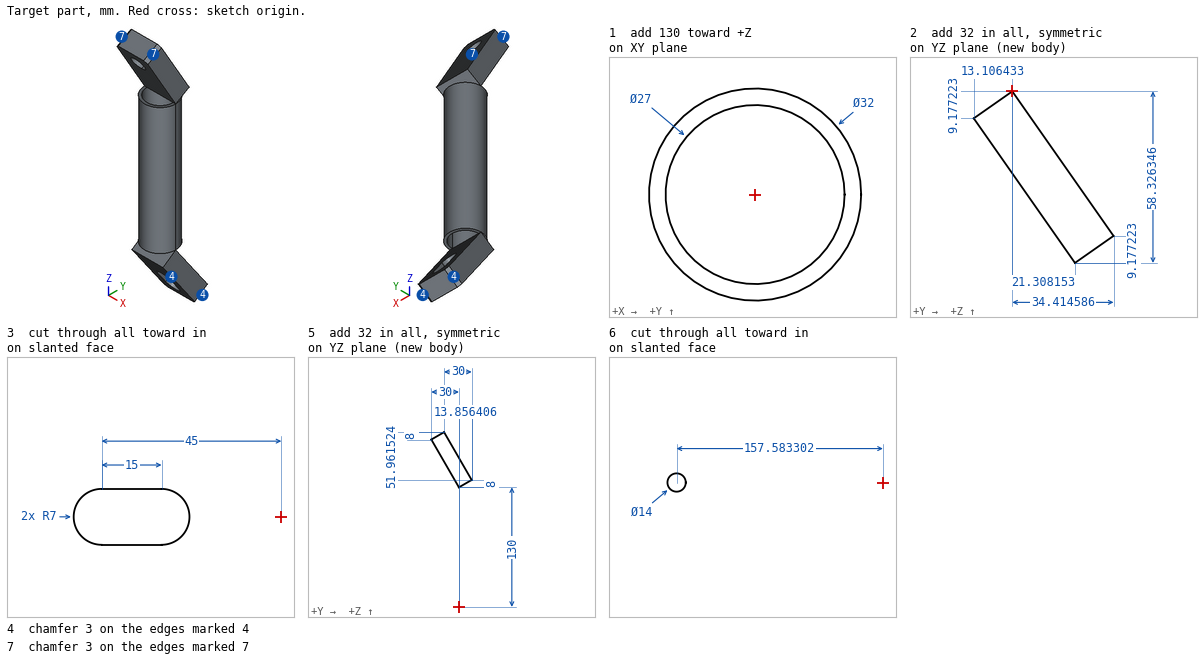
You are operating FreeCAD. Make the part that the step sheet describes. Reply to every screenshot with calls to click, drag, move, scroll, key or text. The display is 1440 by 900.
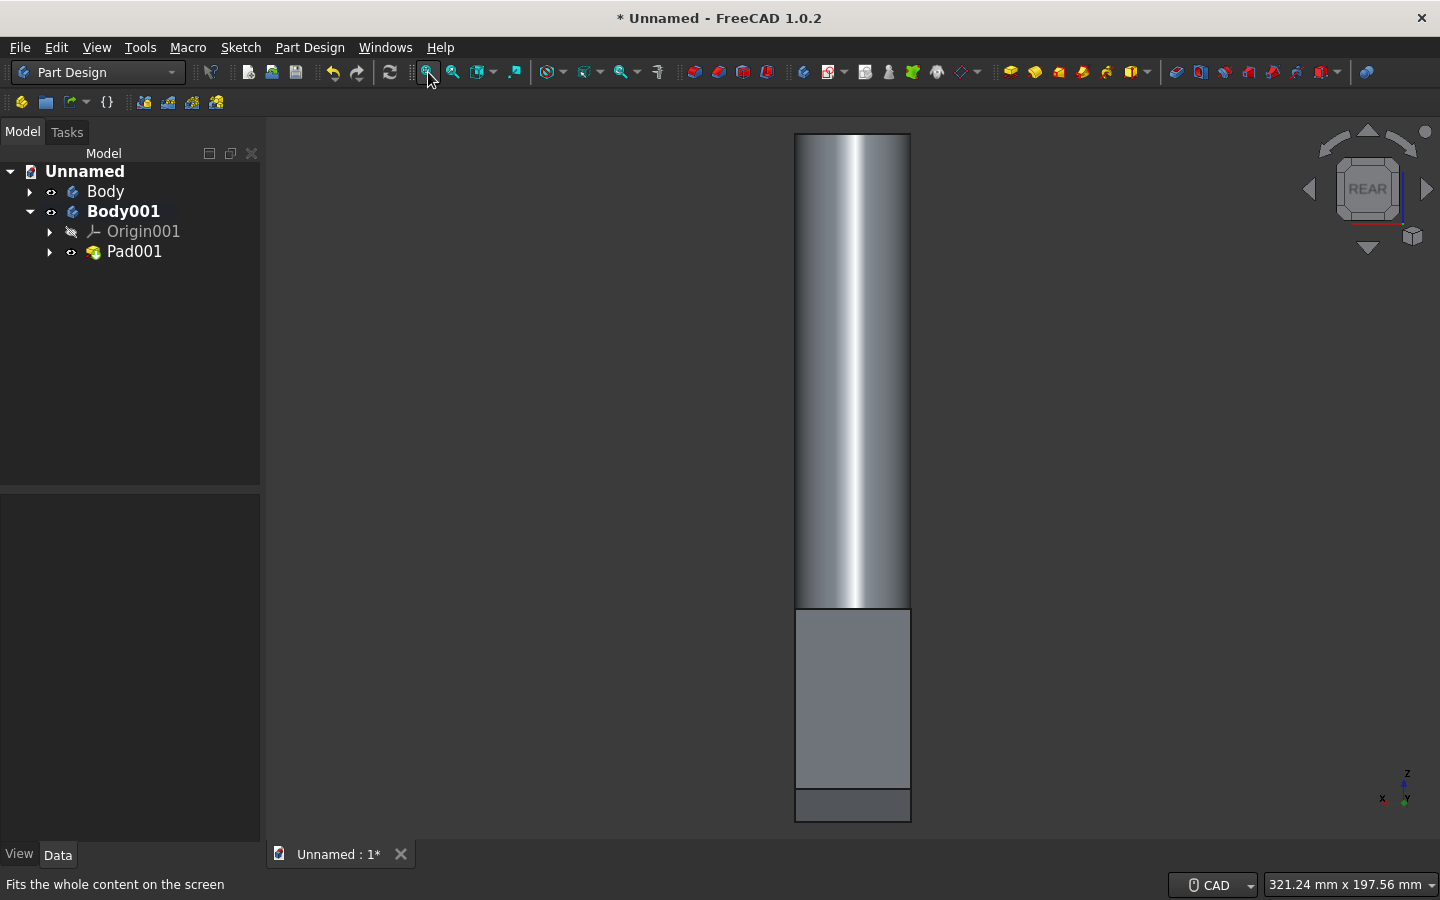
click(853, 723)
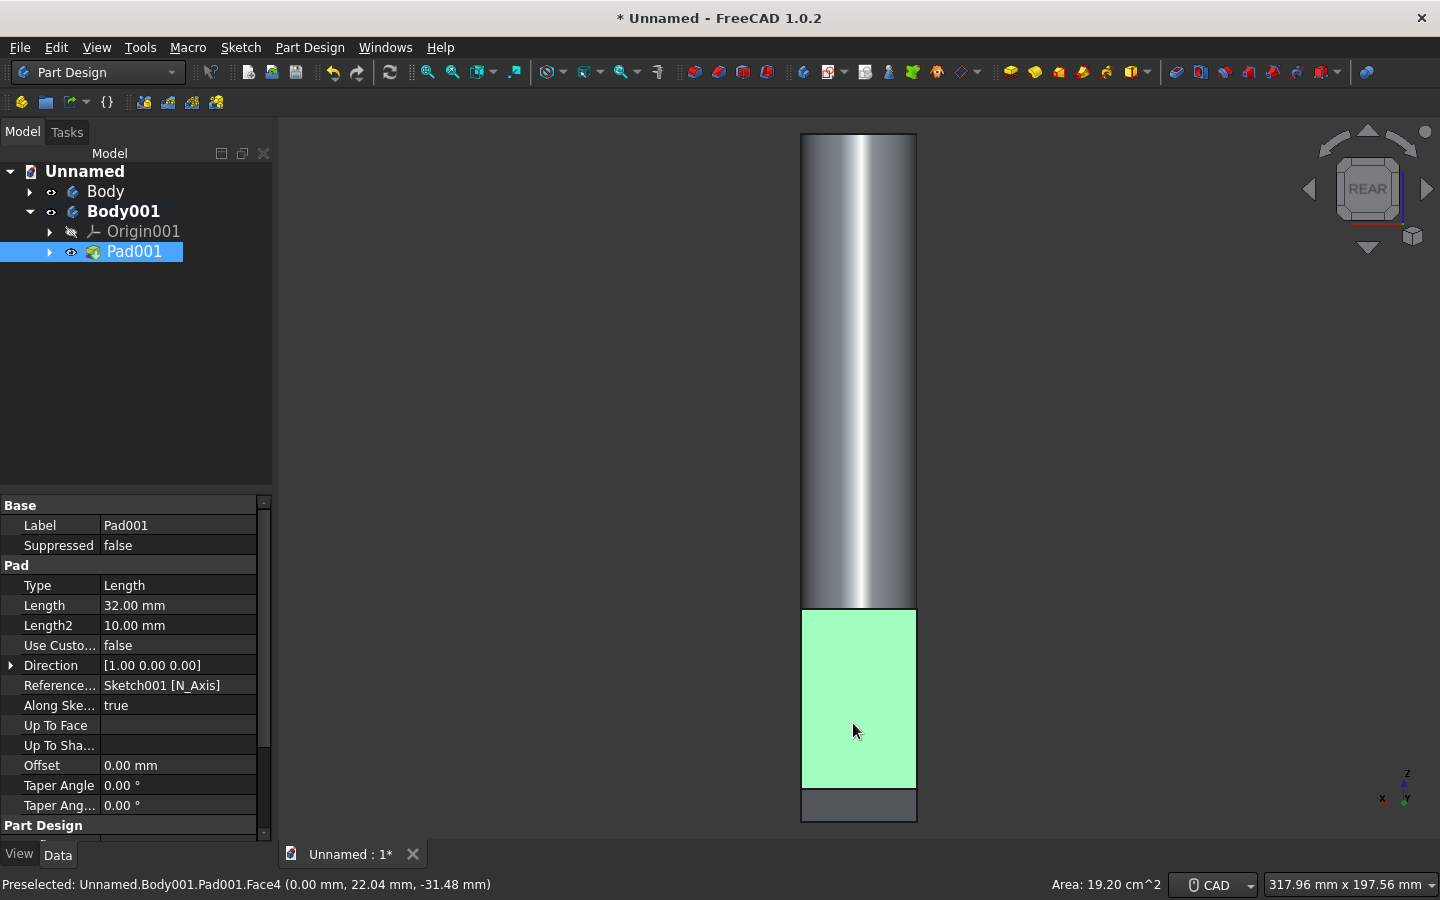
click(828, 72)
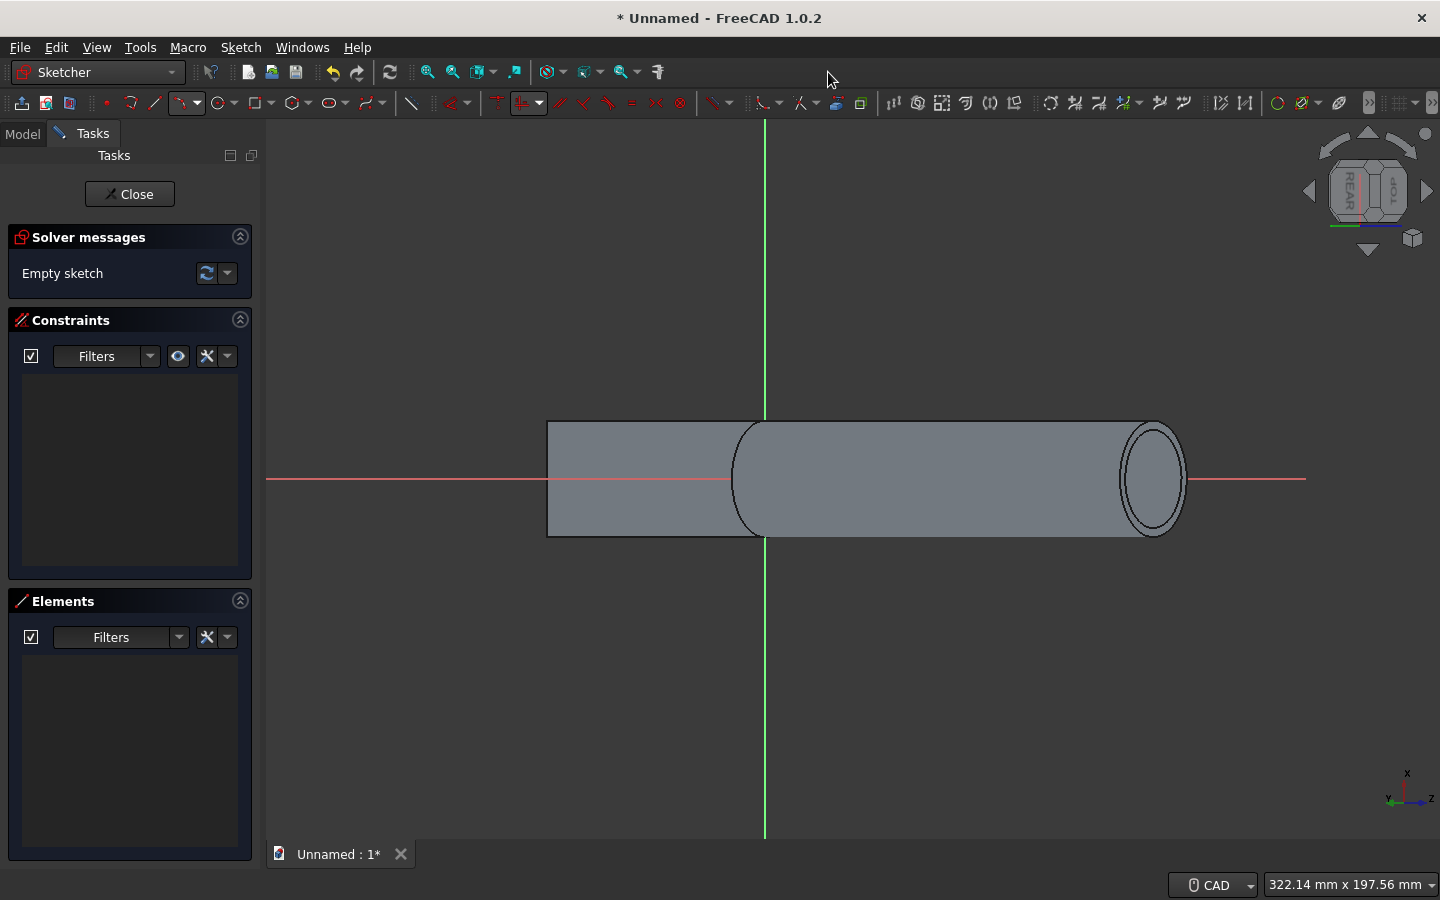
key(q)
key(s)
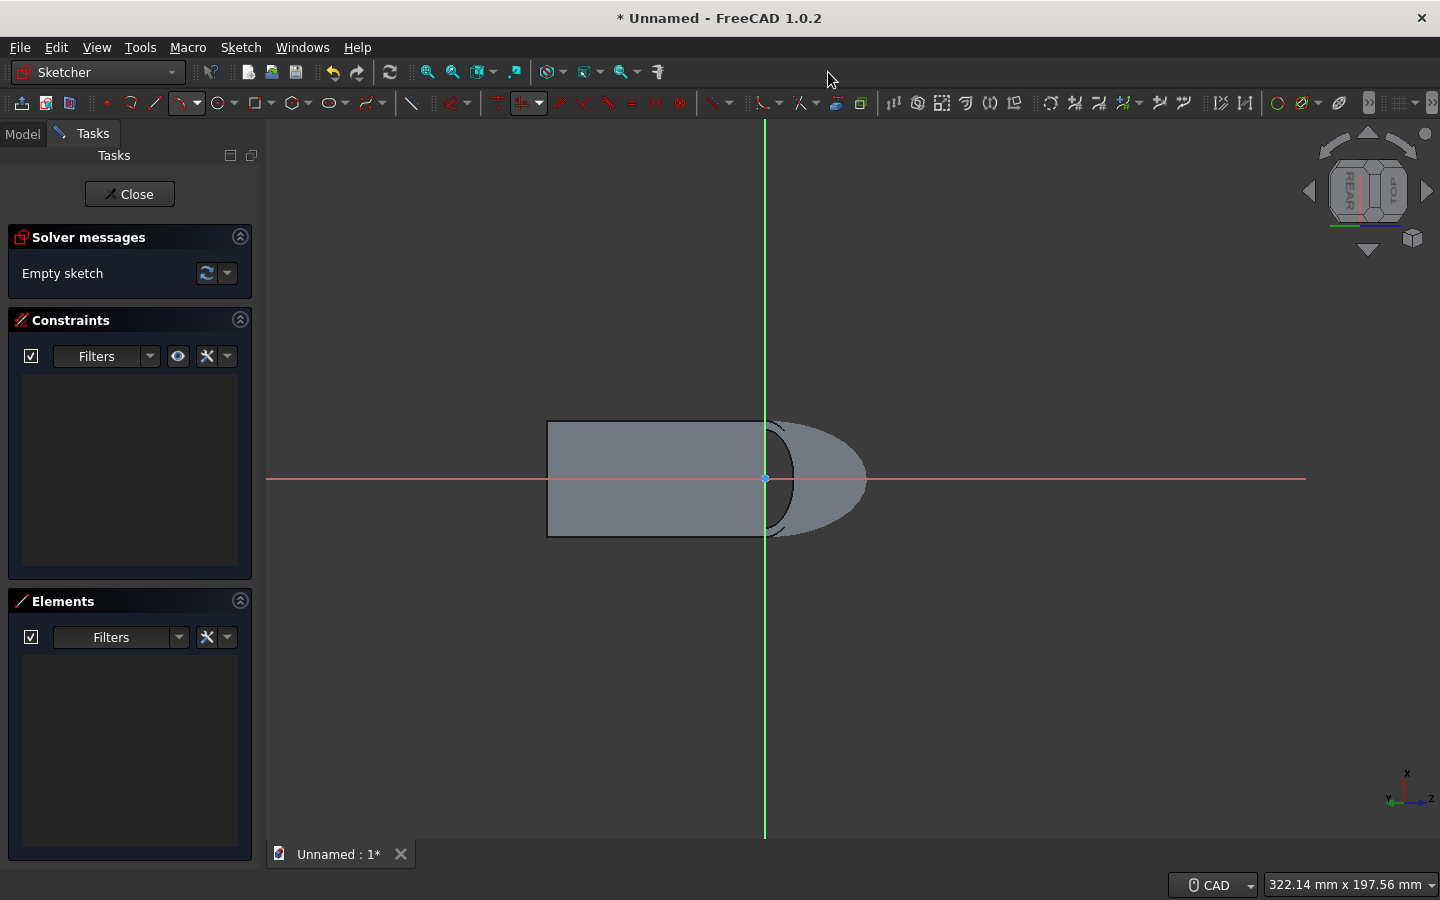
scroll(621, 479, up, 6)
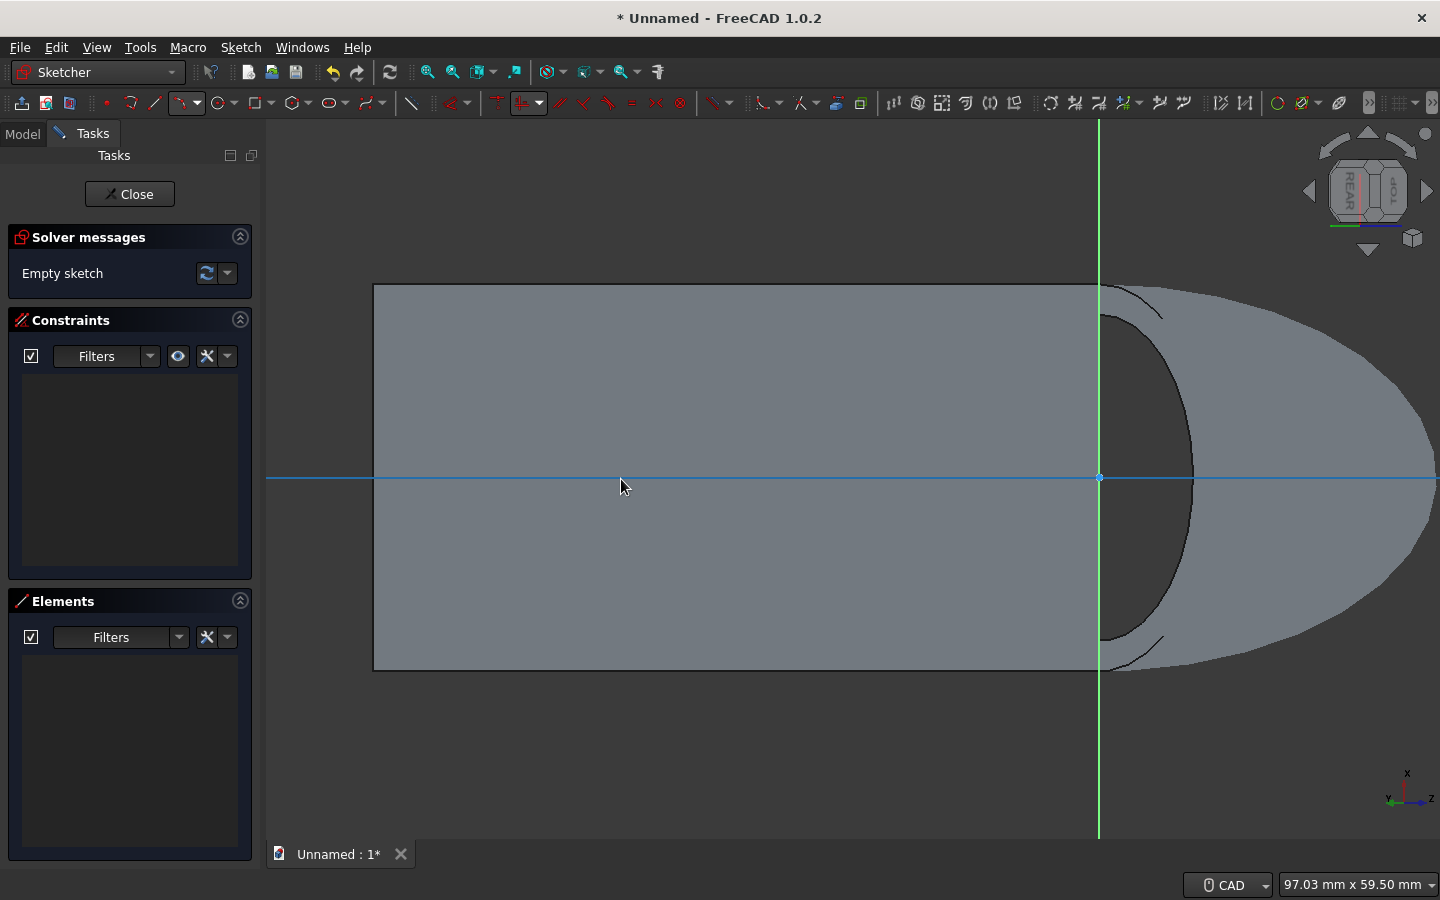
key(g)
key(s)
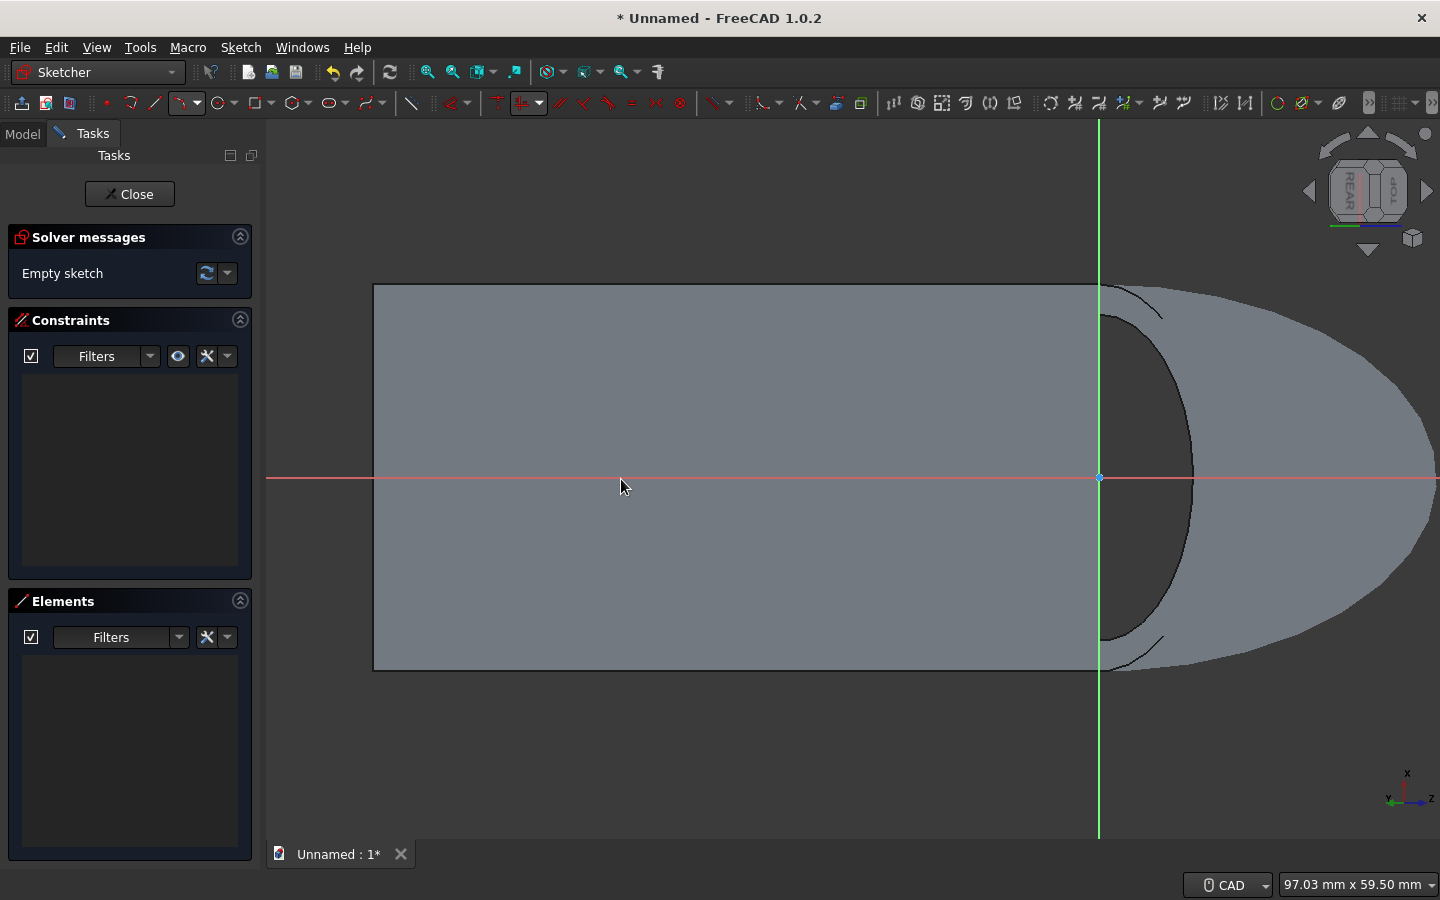
click(555, 478)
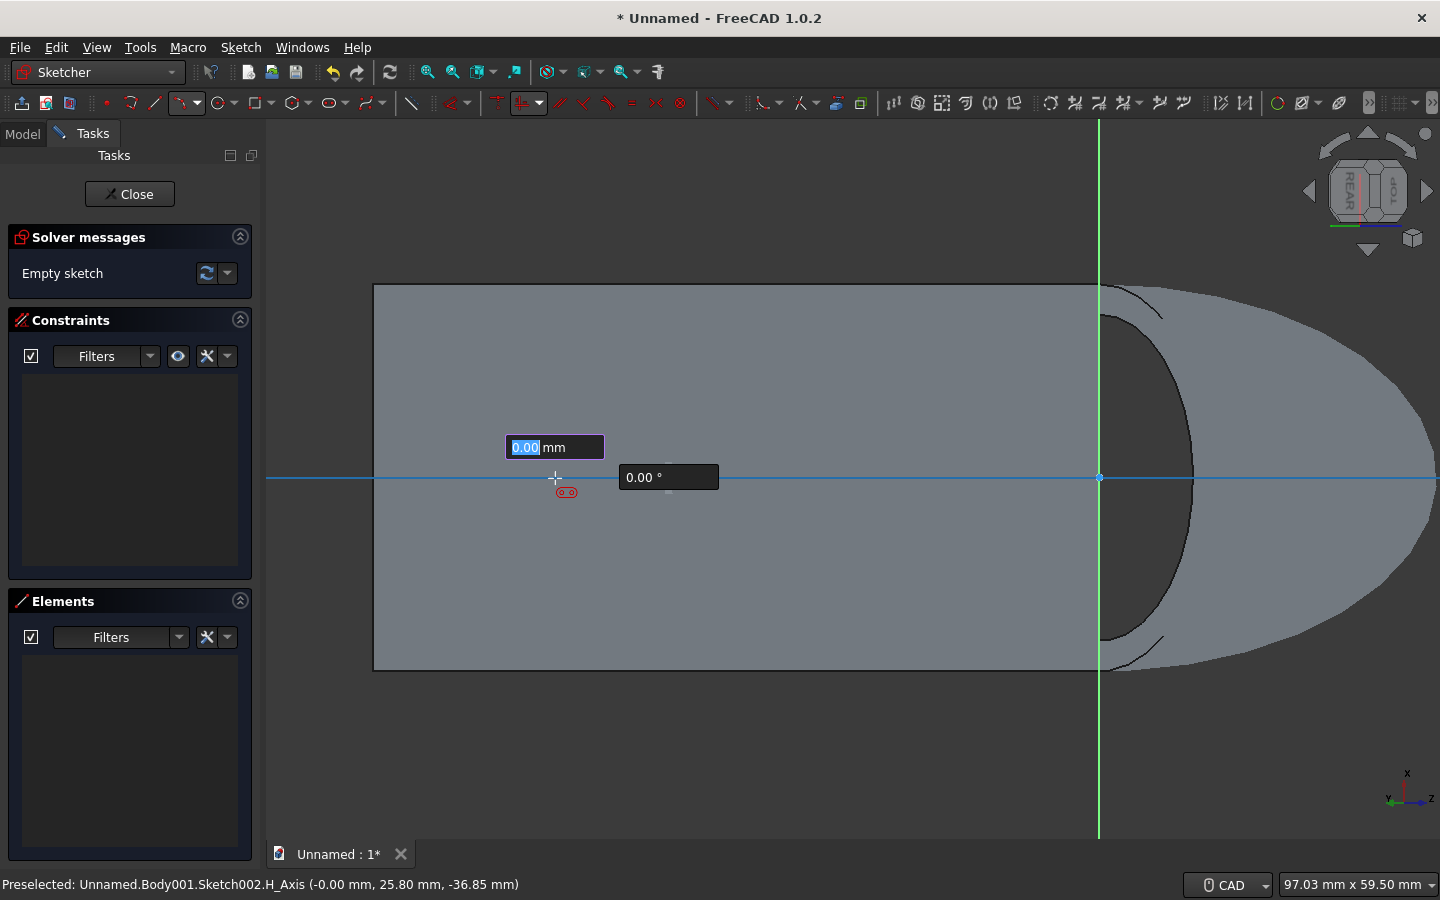
click(736, 469)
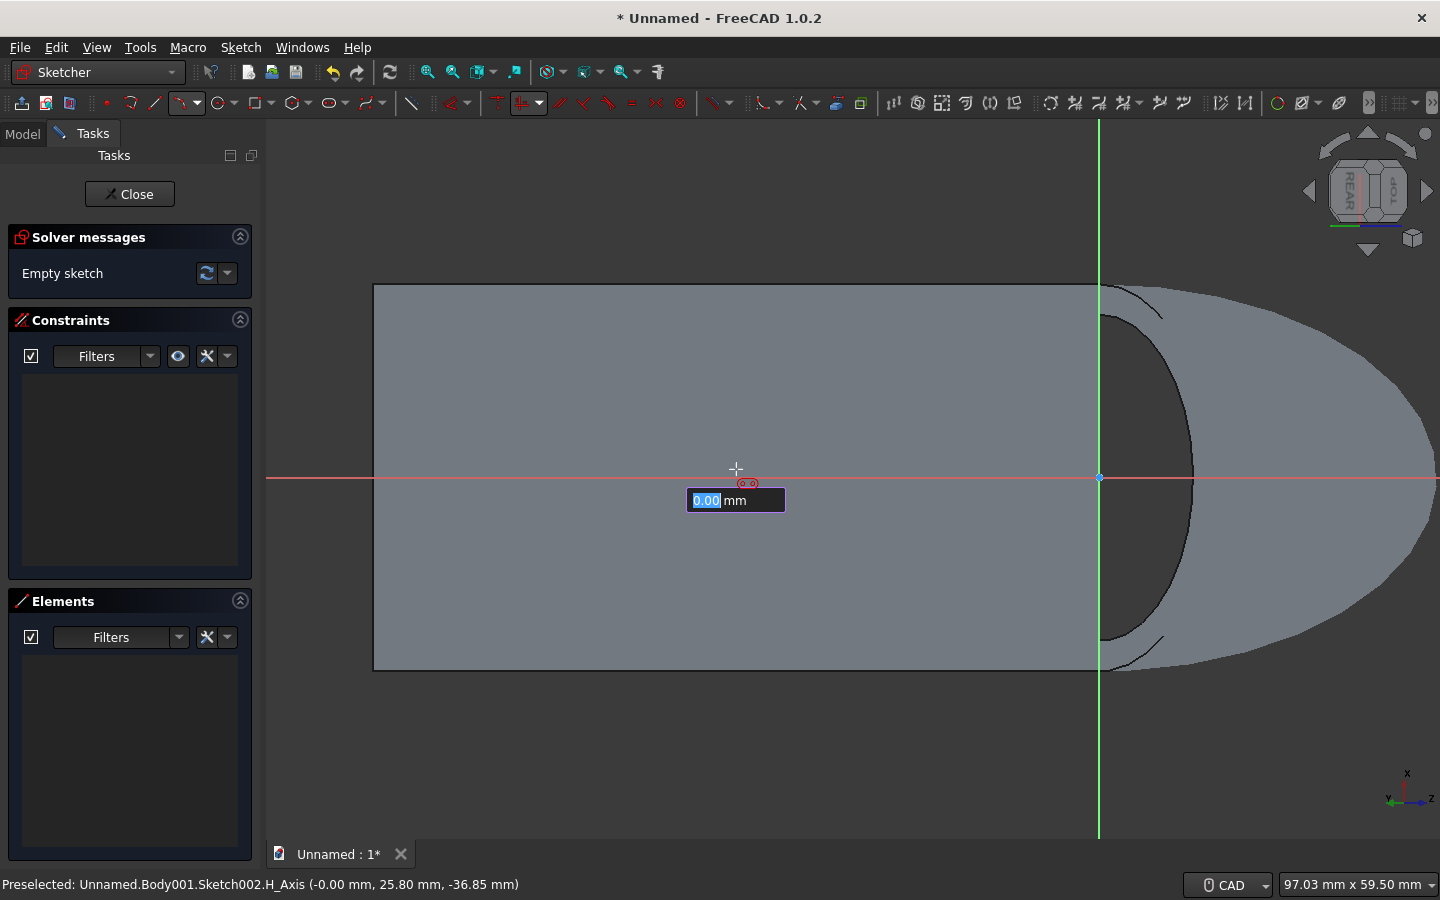
click(646, 393)
key(Escape)